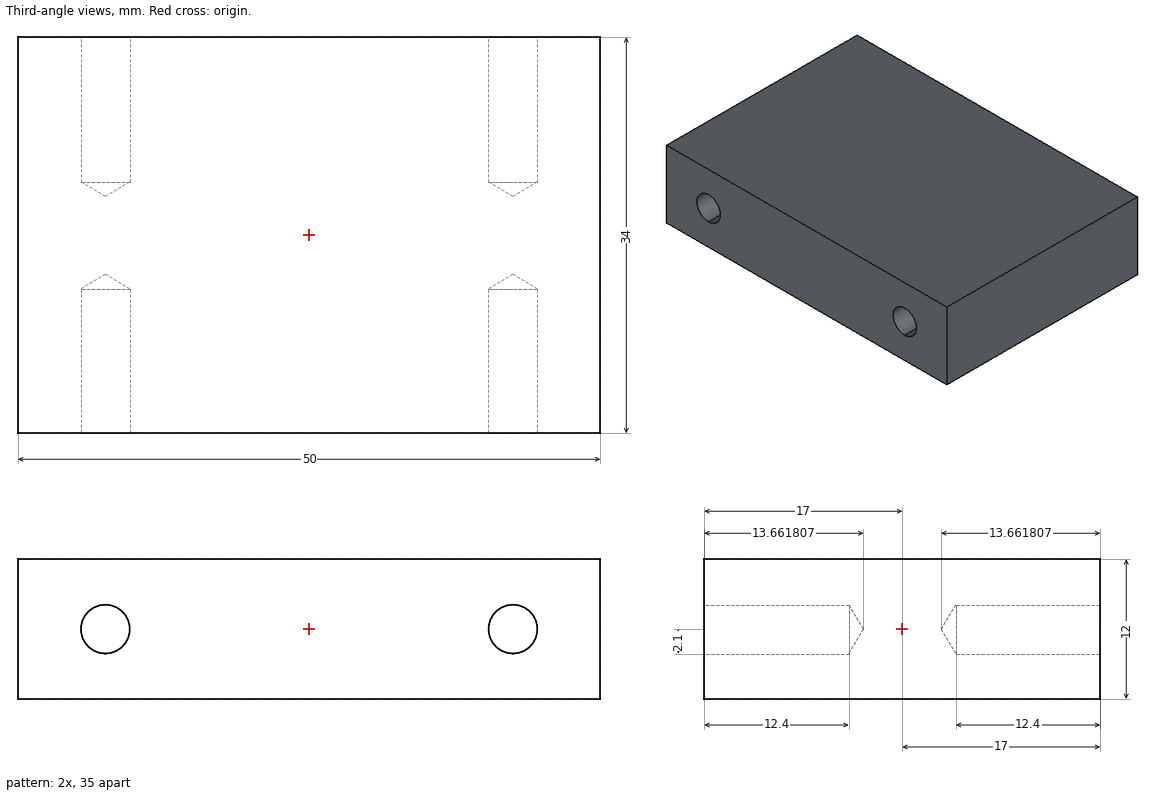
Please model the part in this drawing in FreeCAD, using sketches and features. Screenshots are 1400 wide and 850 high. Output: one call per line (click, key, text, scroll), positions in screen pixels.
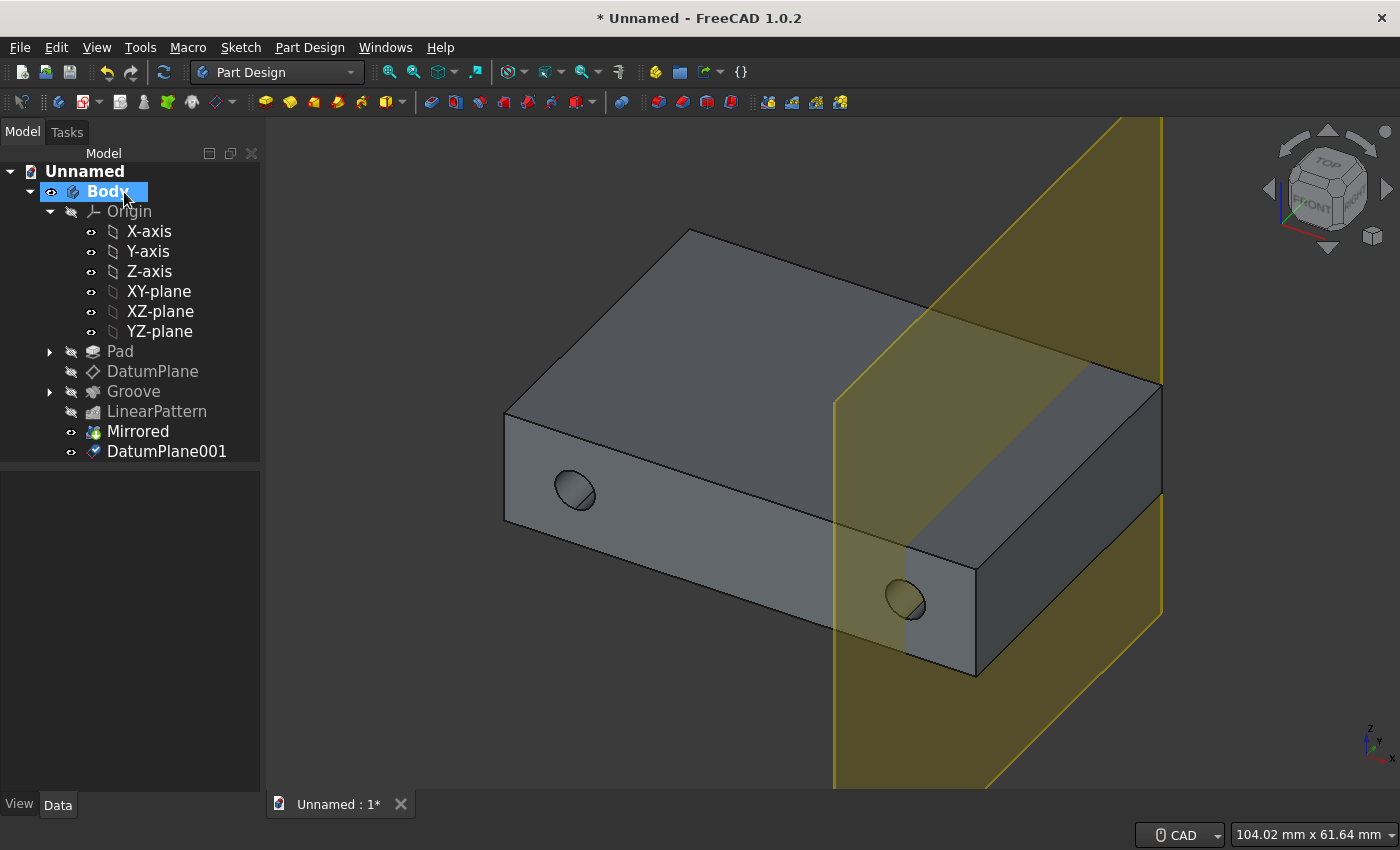
click(116, 452)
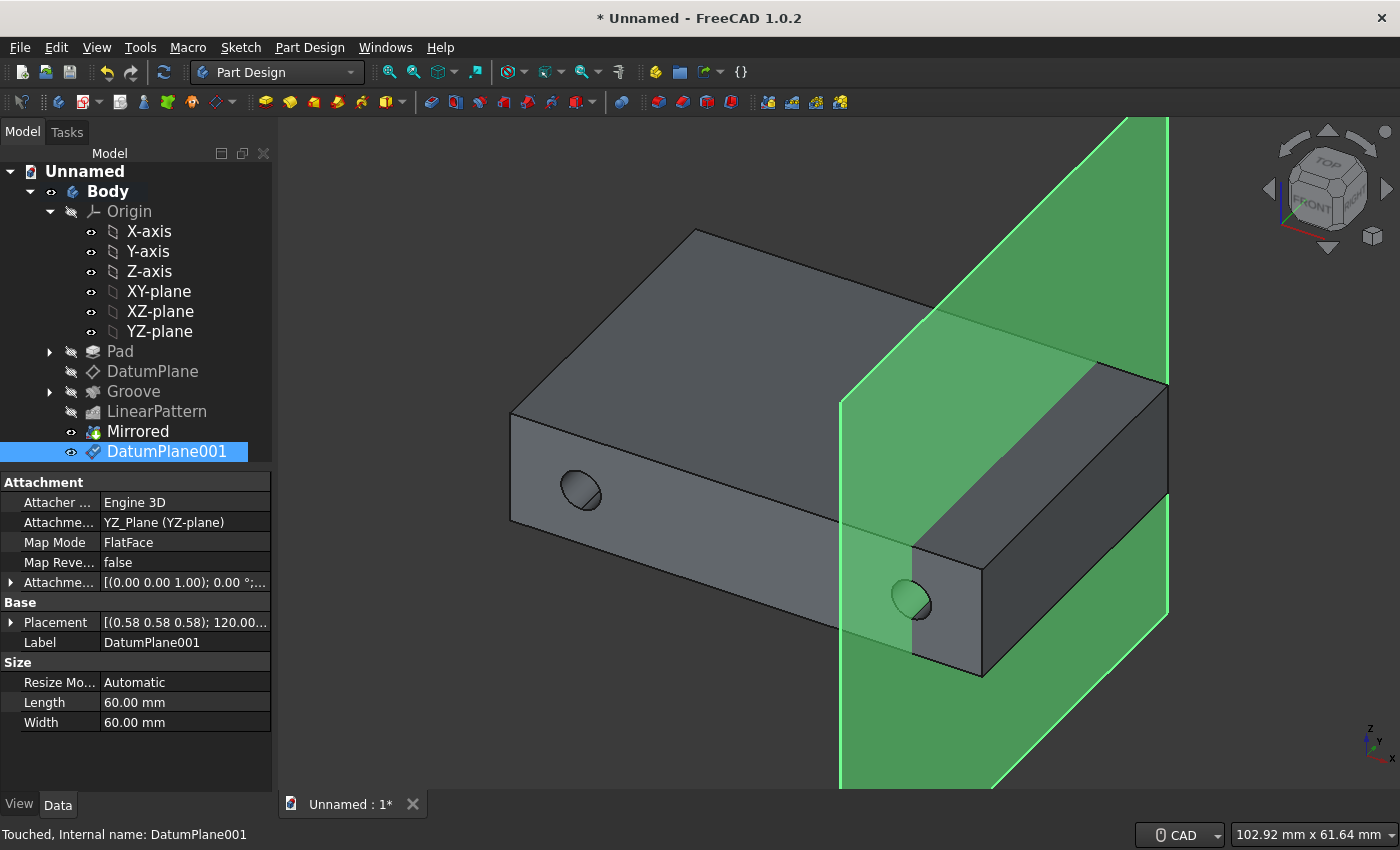
click(84, 102)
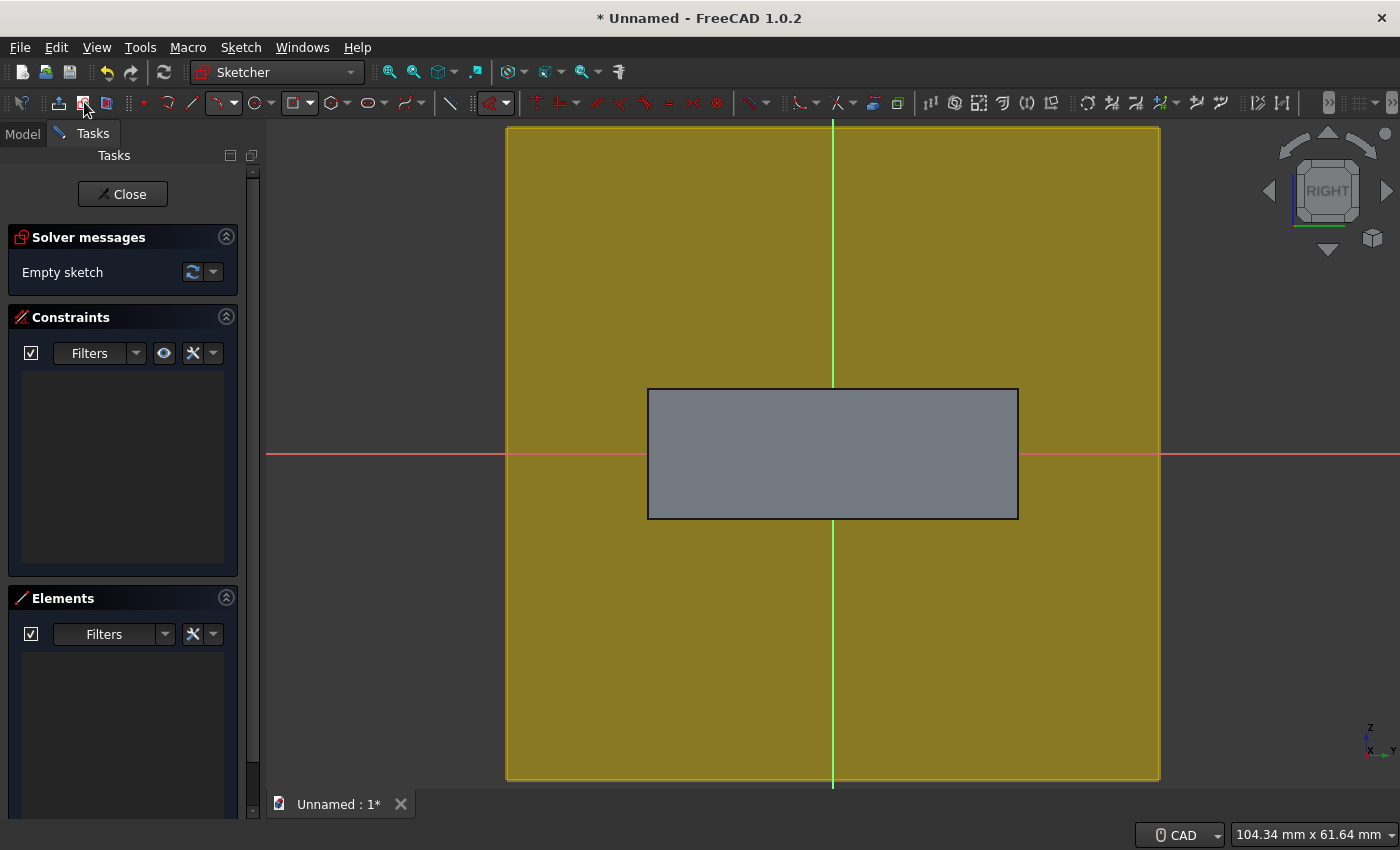
click(108, 104)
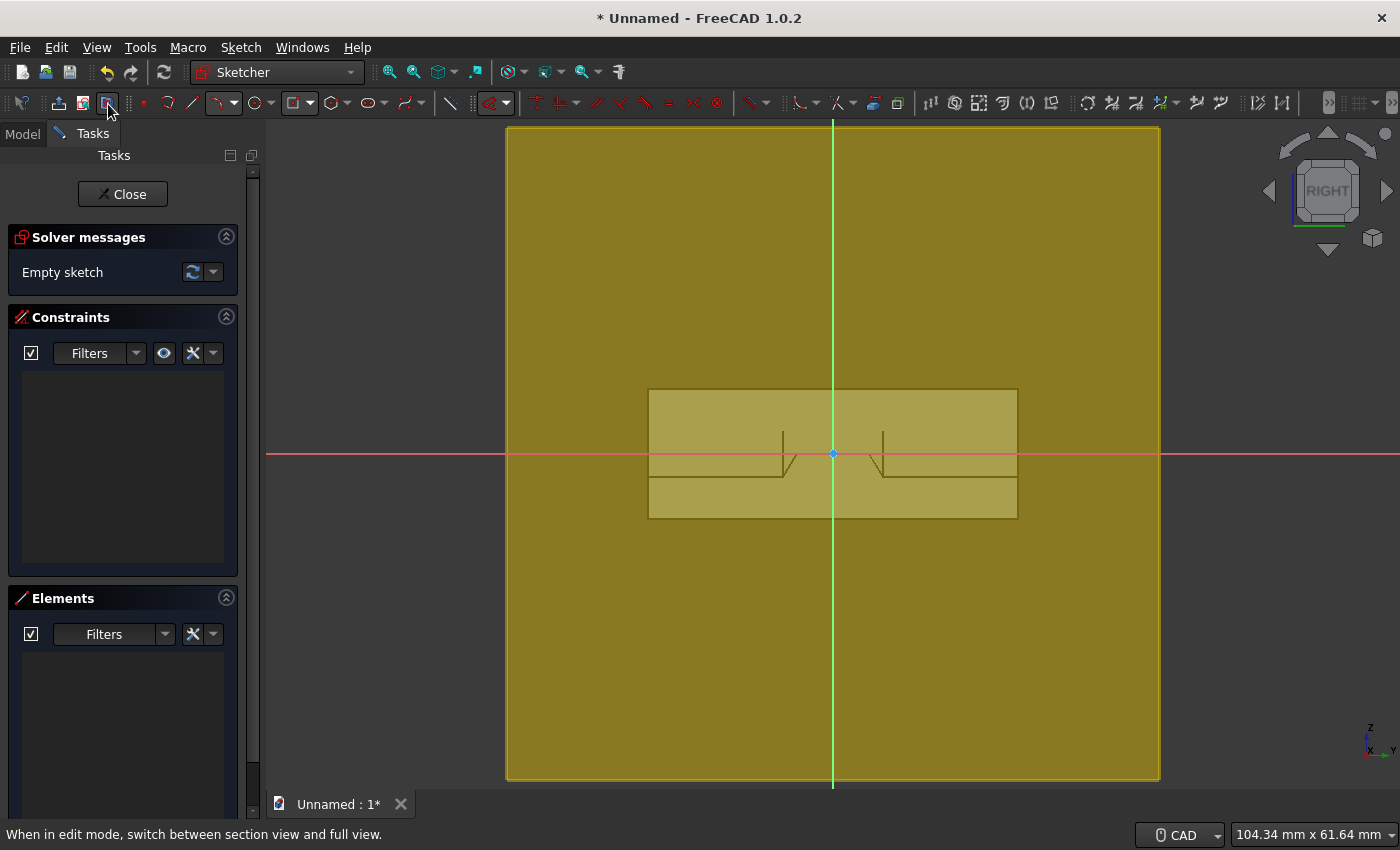
scroll(995, 470, up, 6)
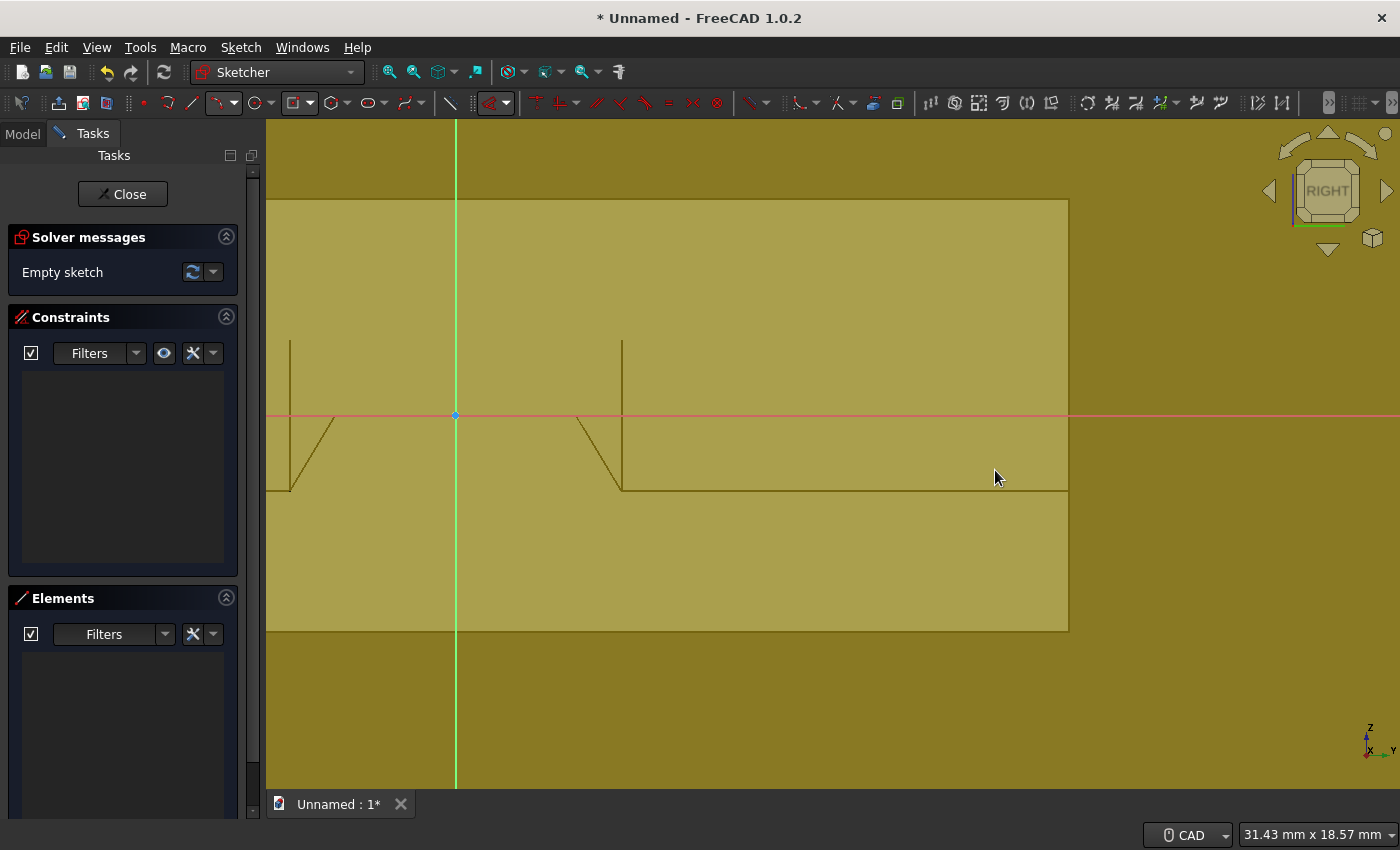
key(g)
key(m)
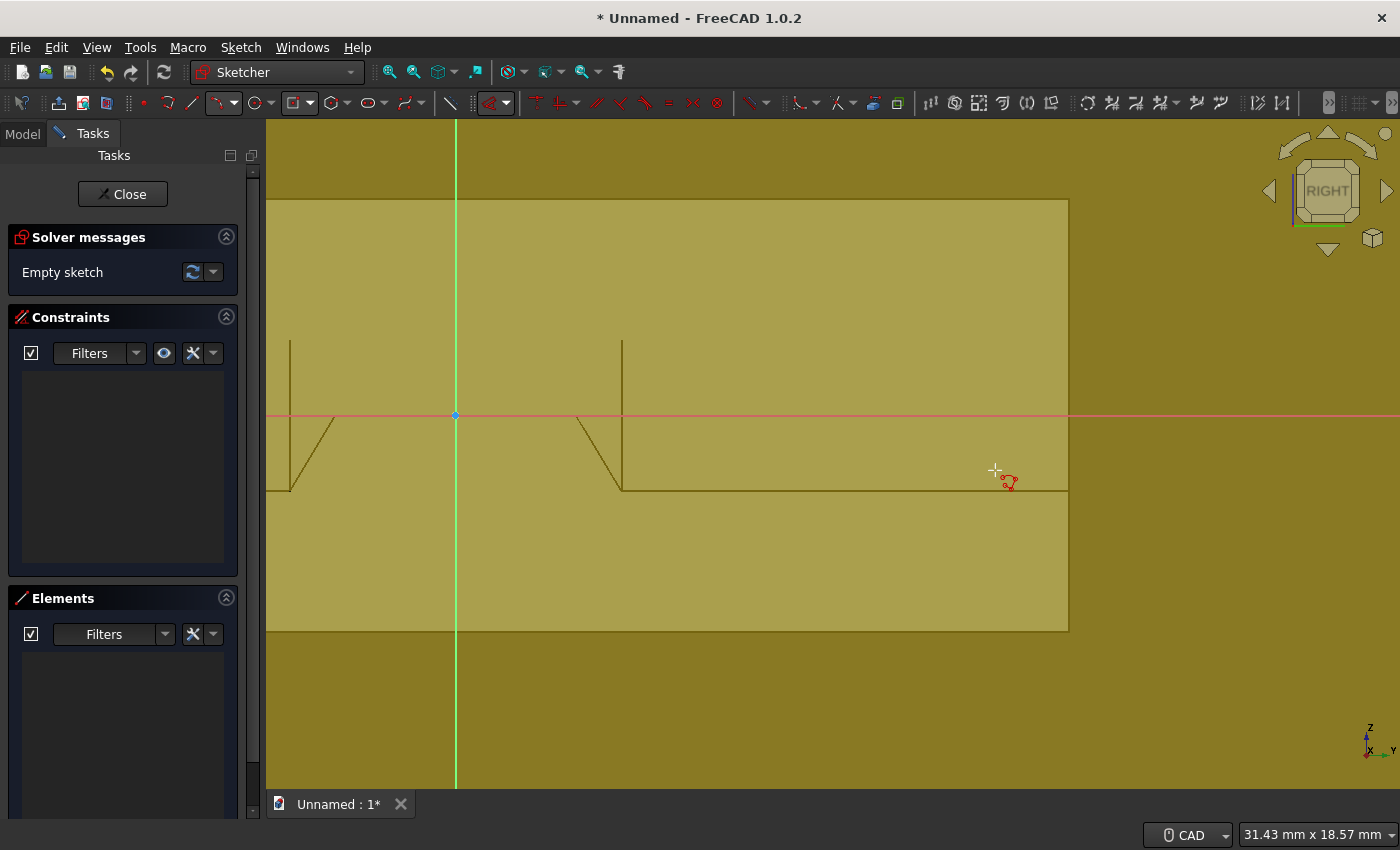
click(576, 416)
click(622, 491)
click(1069, 491)
click(1069, 425)
click(576, 416)
key(Escape)
key(Escape)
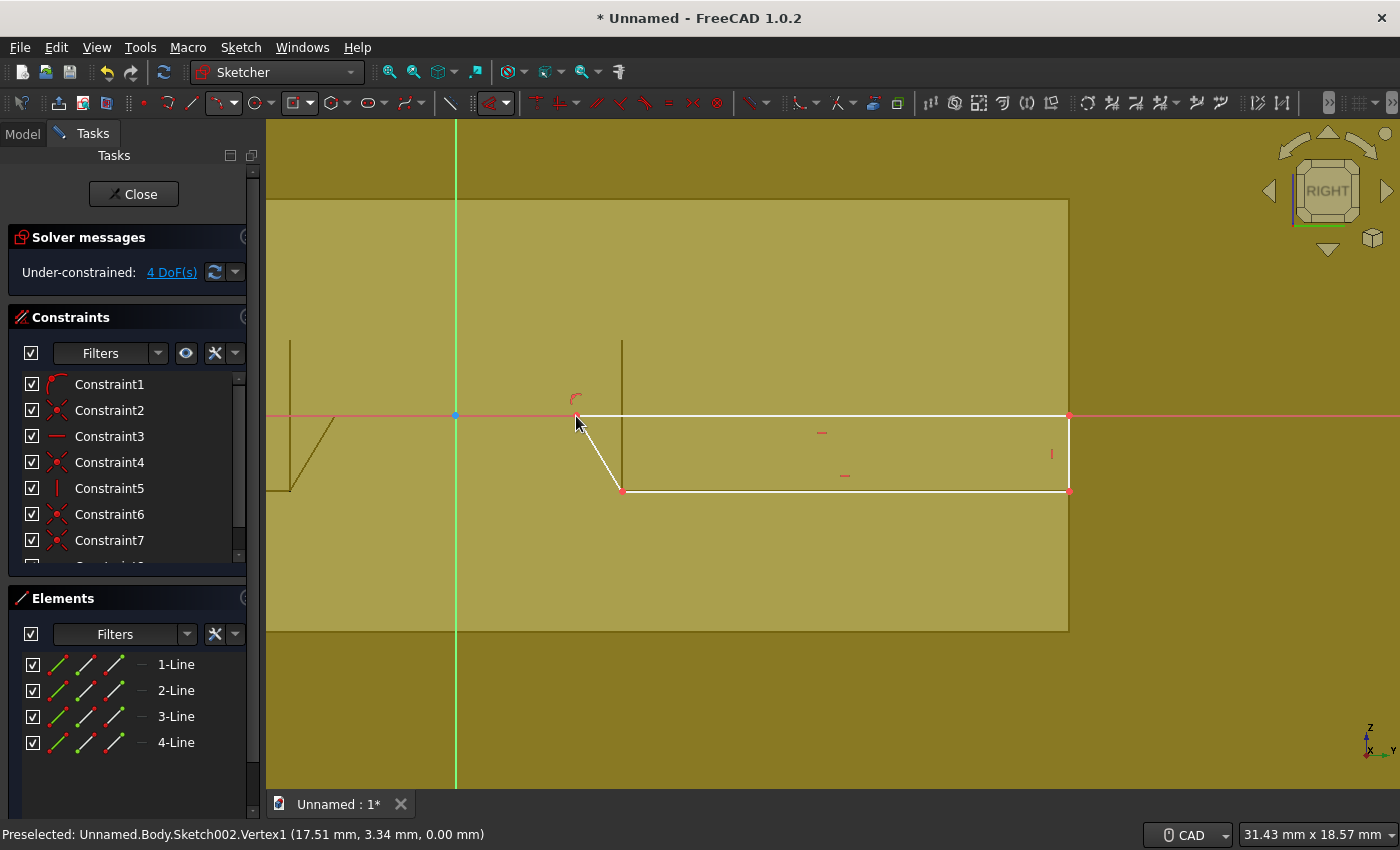
click(1069, 469)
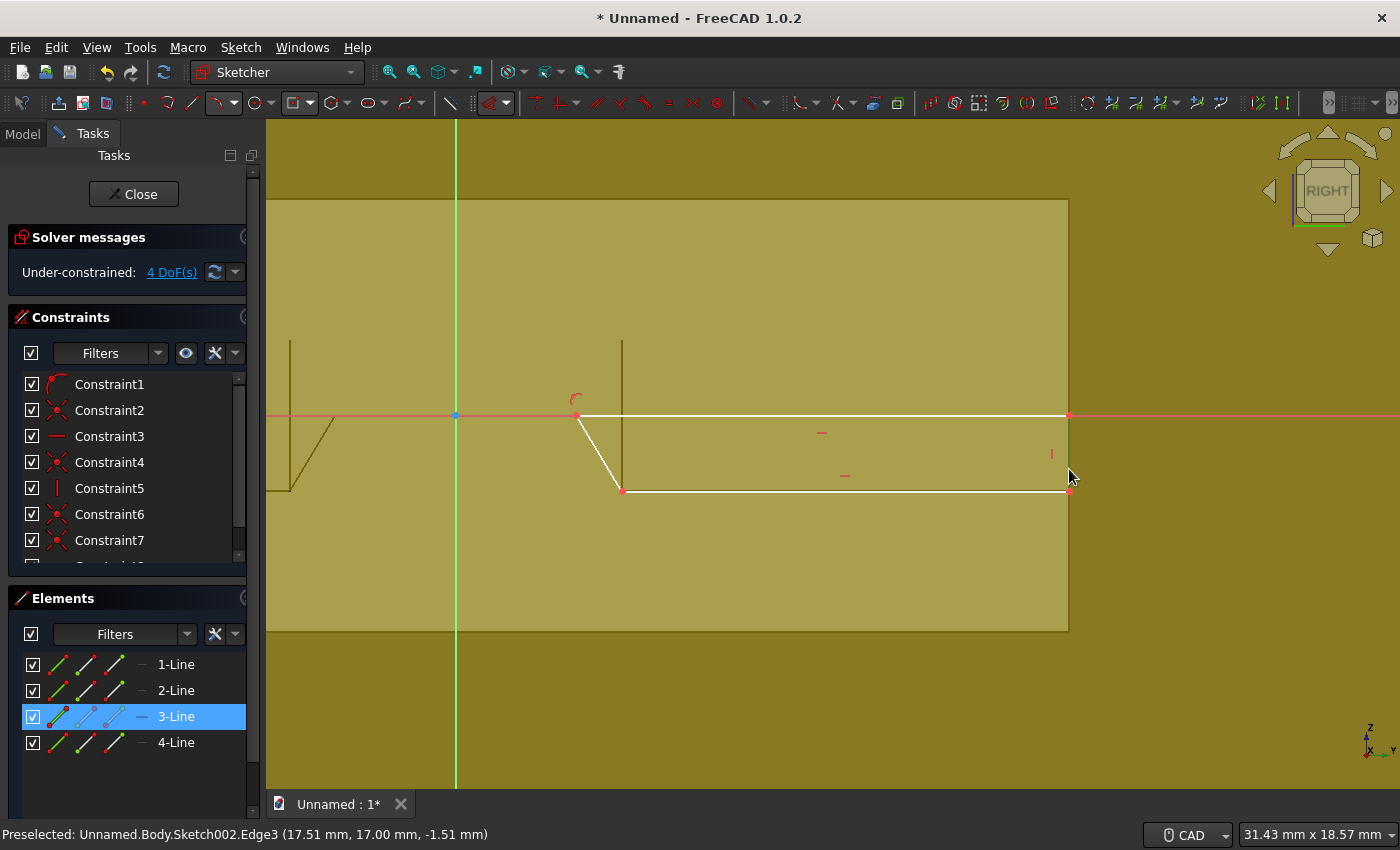
key(i)